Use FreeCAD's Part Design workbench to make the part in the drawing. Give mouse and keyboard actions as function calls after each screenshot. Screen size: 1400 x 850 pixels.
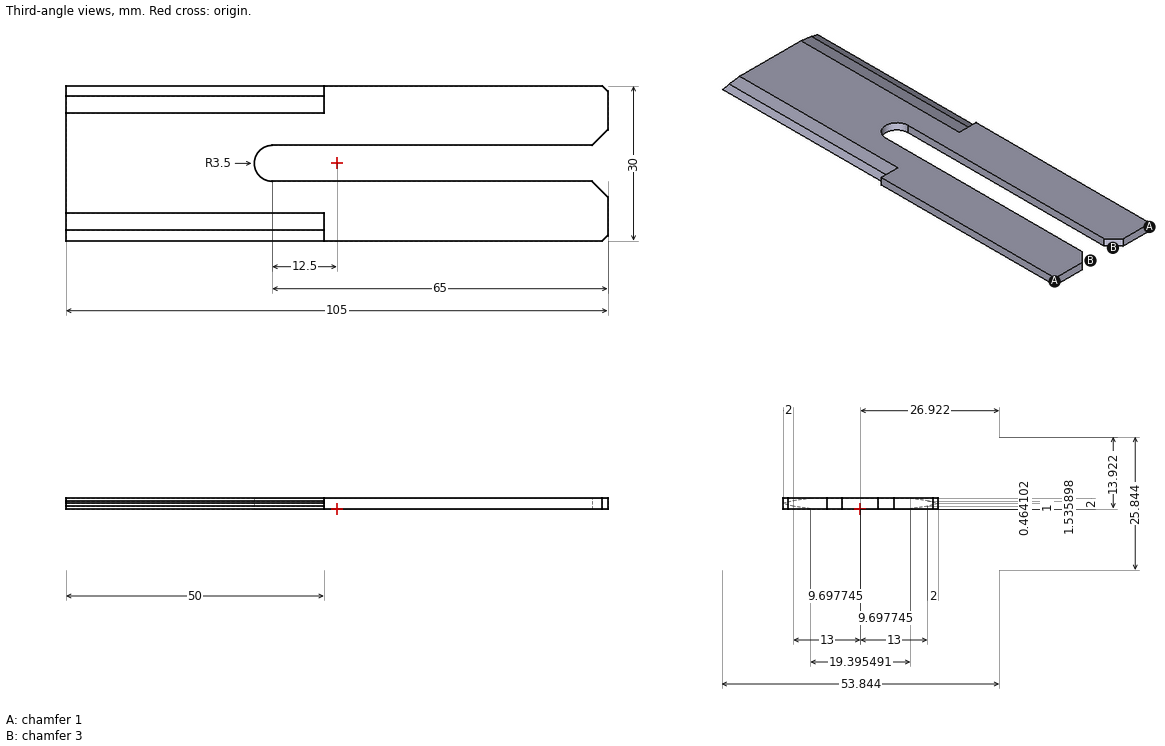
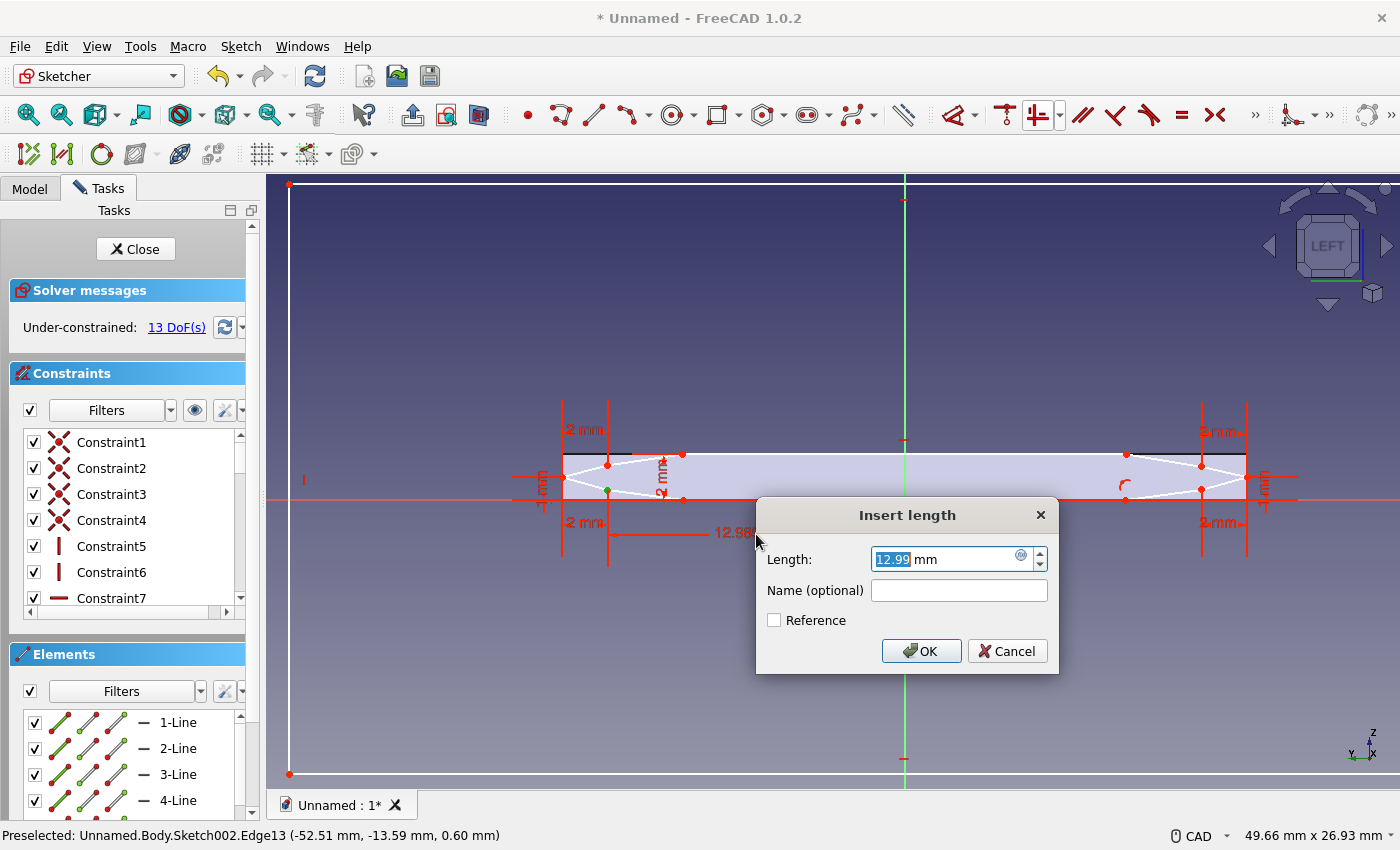
text(13)
key(Return)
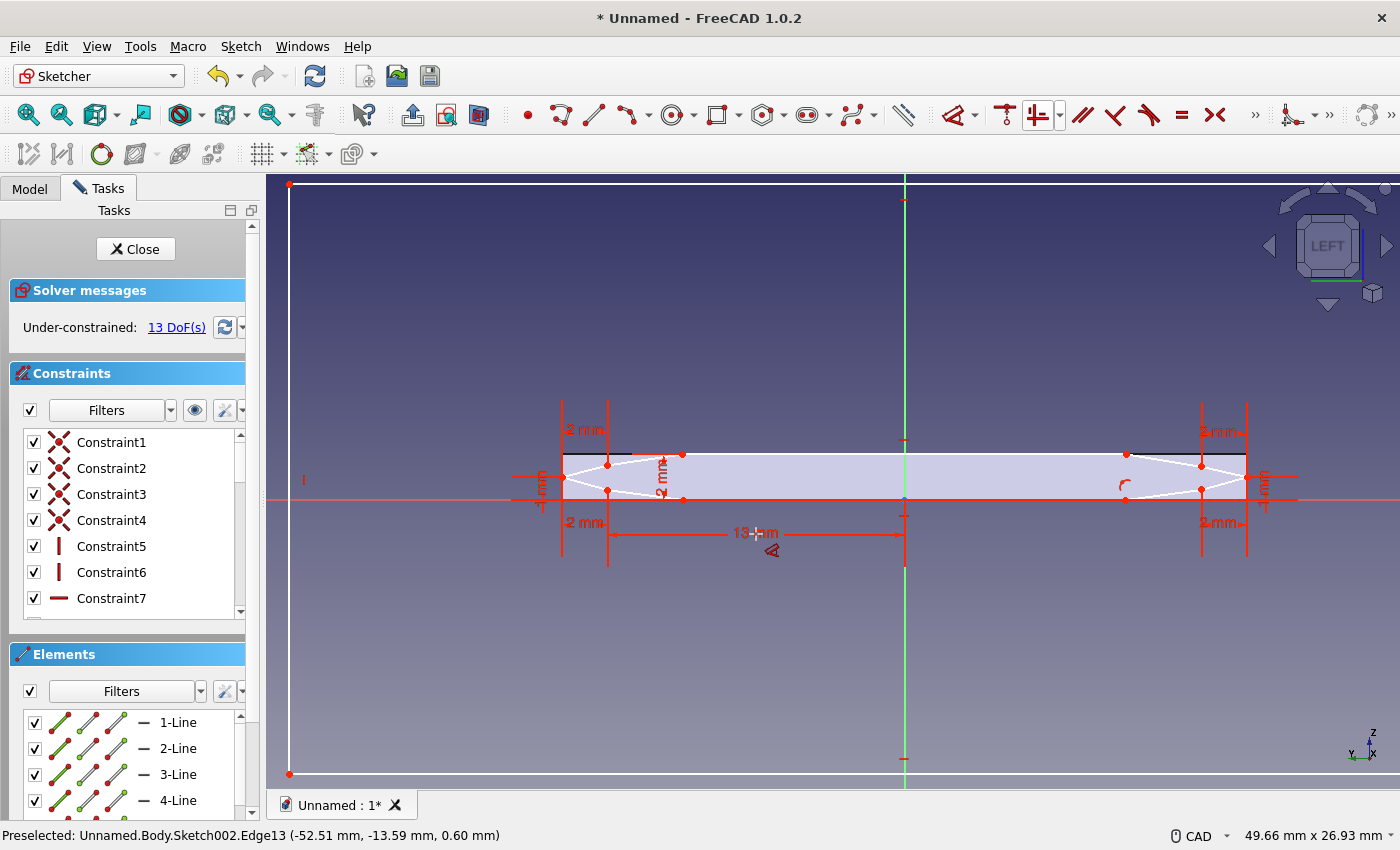
click(1202, 467)
click(1053, 534)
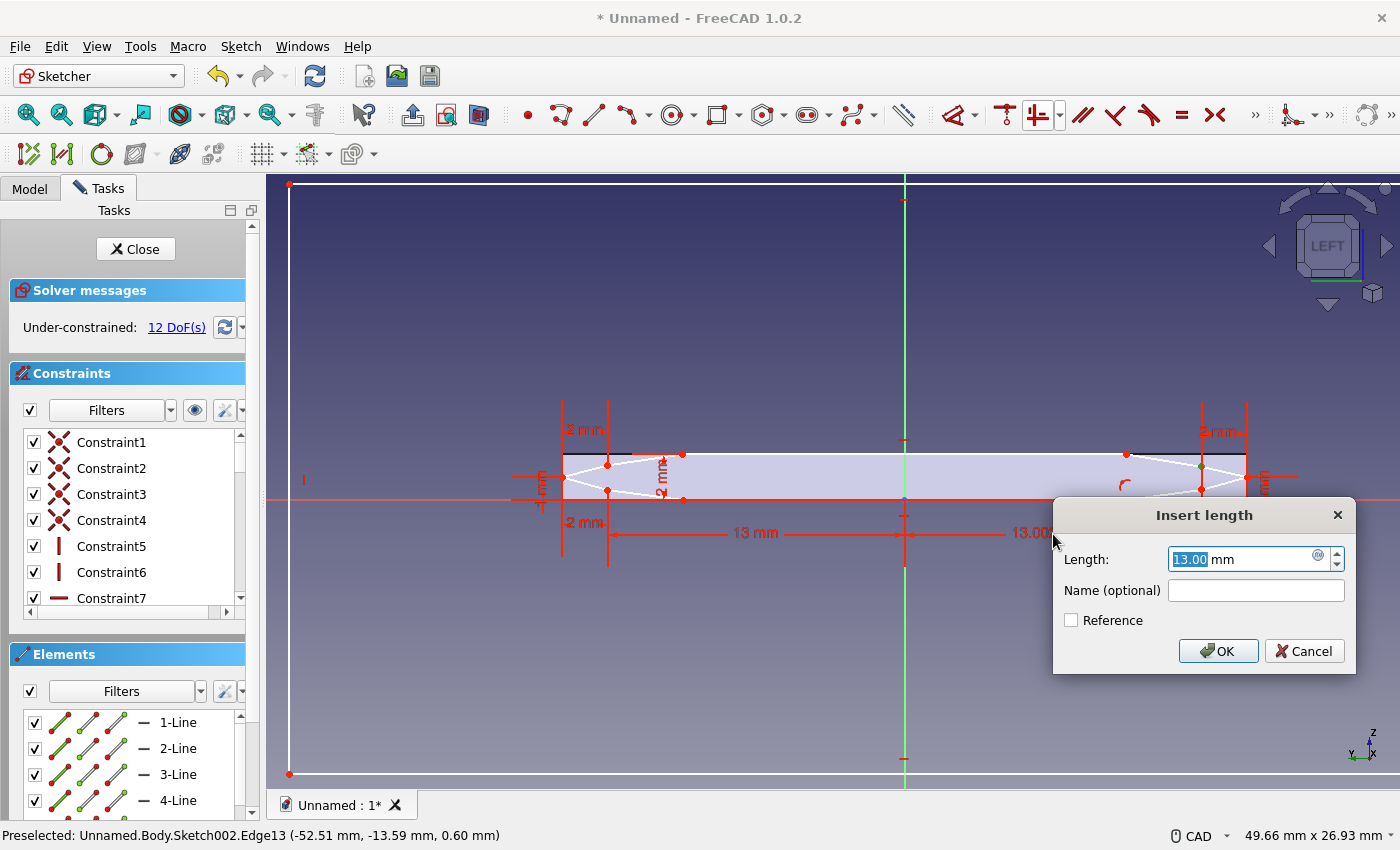
text(13)
key(Return)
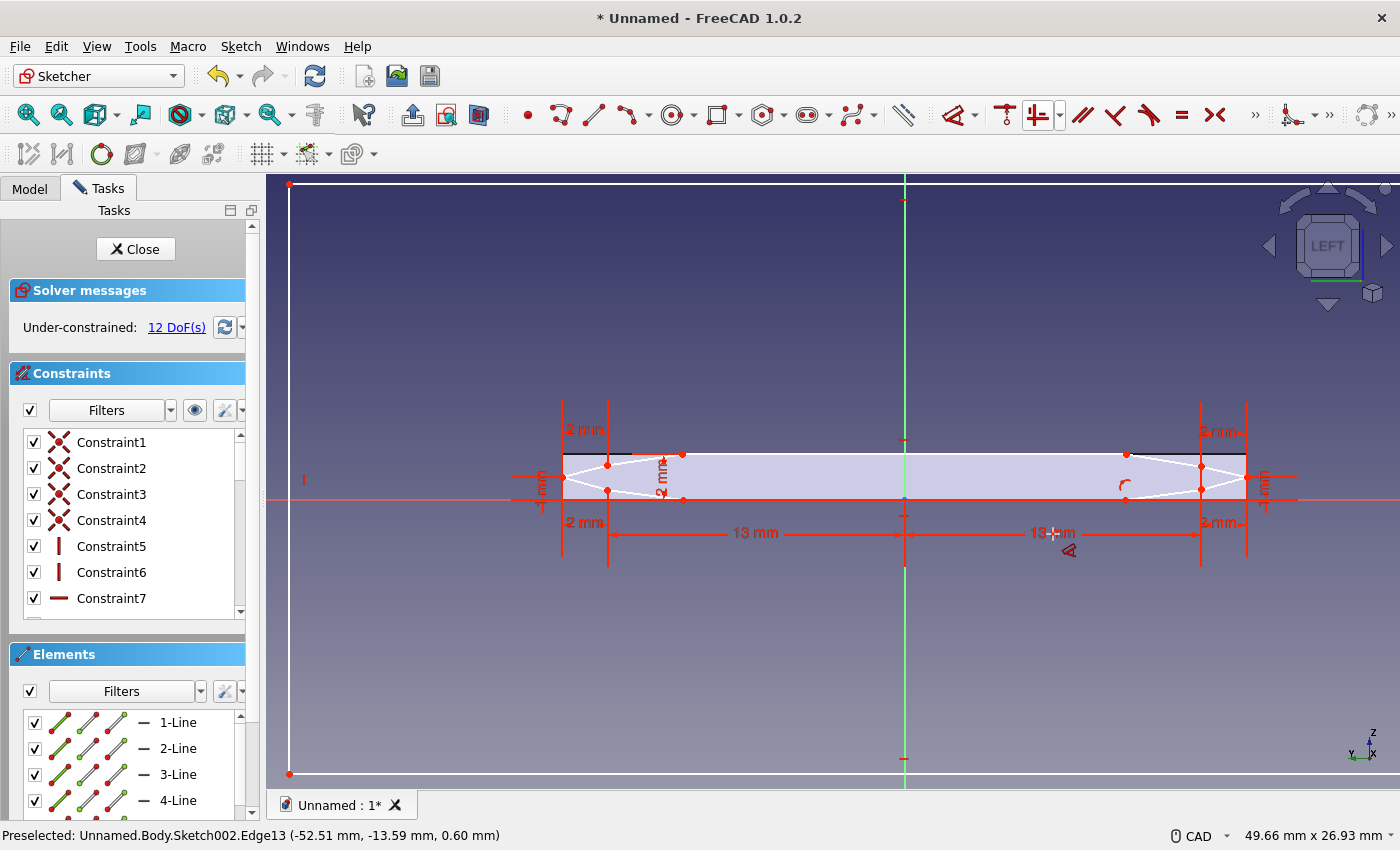
scroll(594, 487, down, 3)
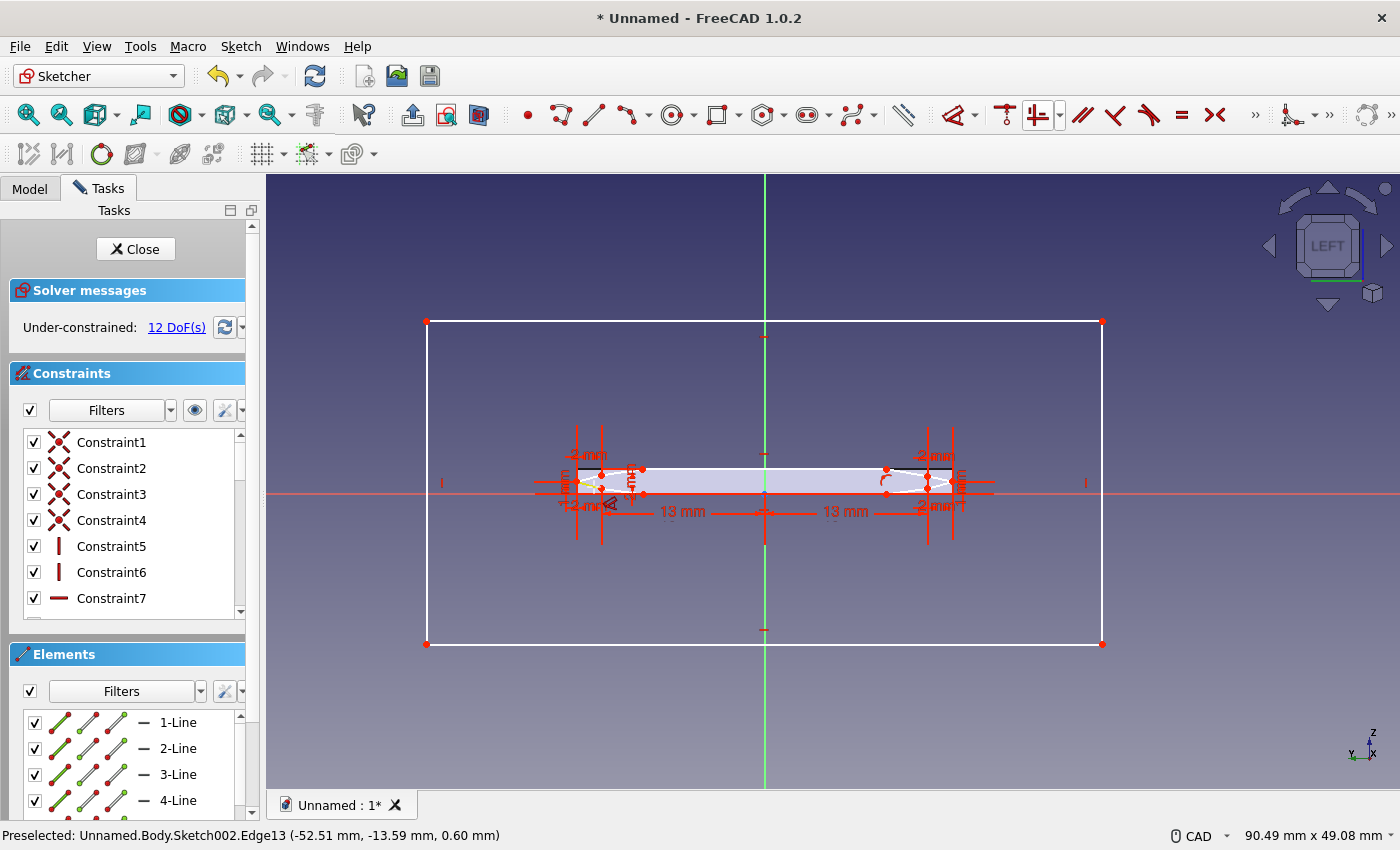
click(427, 418)
click(393, 409)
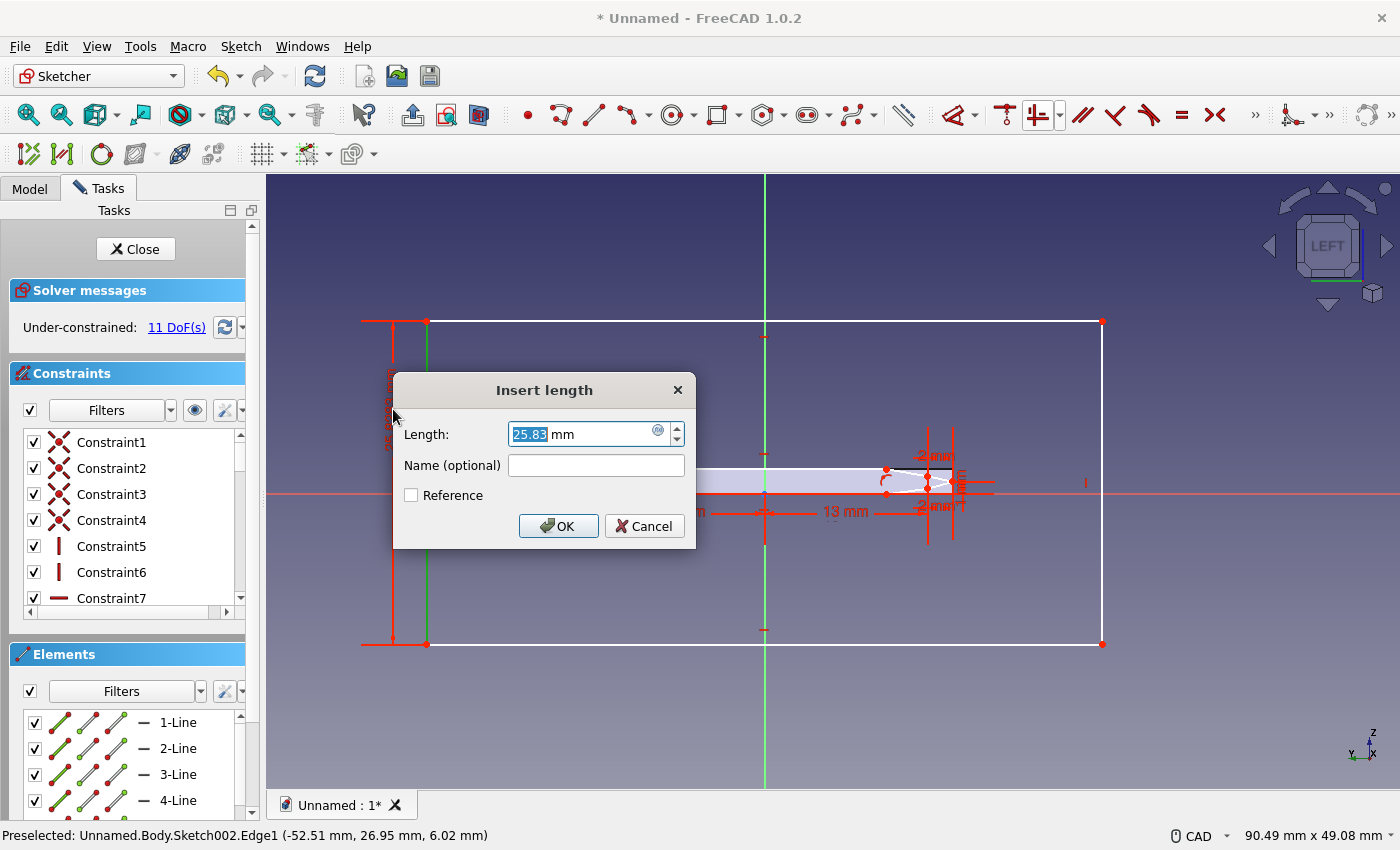
text(25.844)
key(Return)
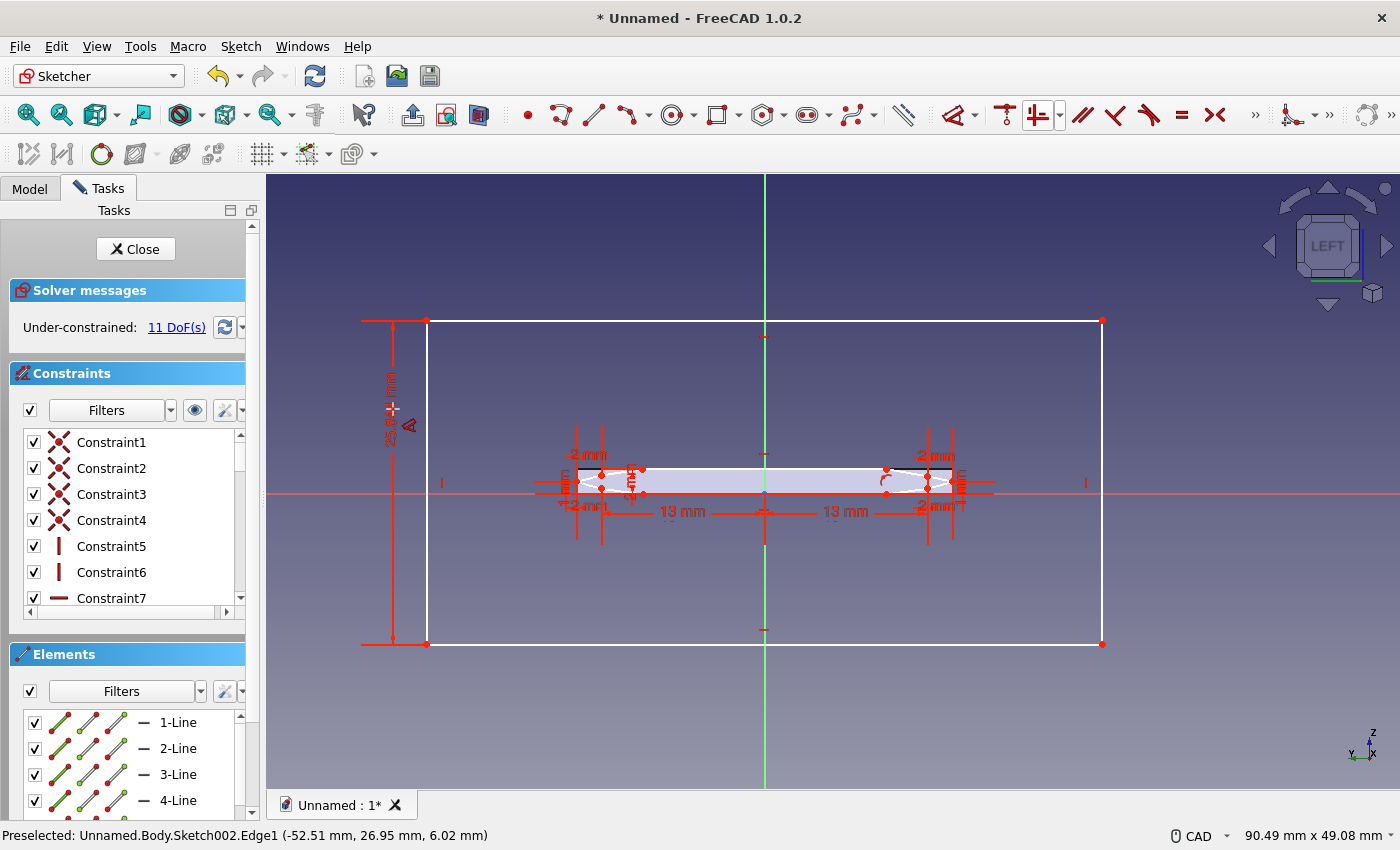
click(629, 645)
click(609, 679)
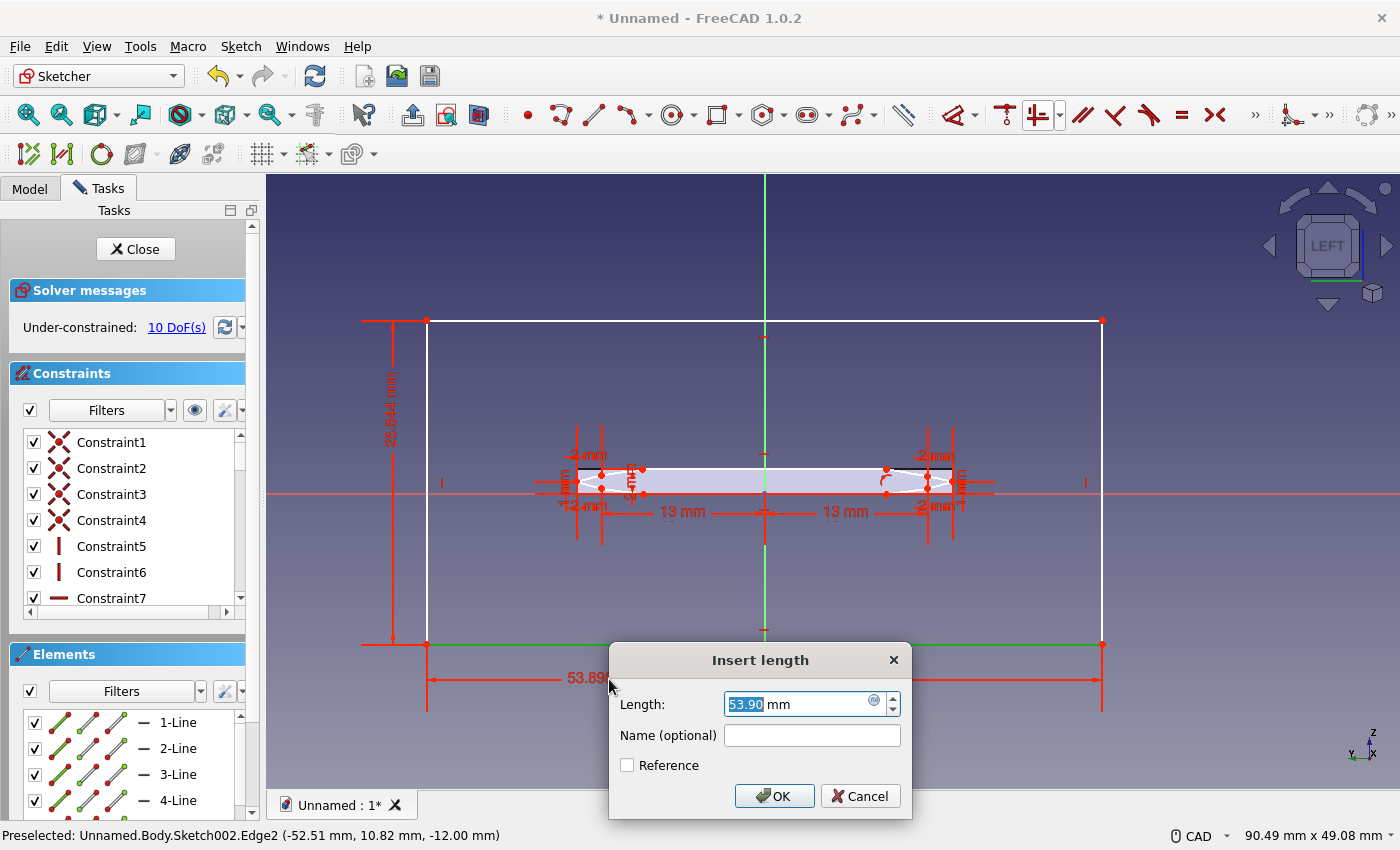
text(53.844)
key(Return)